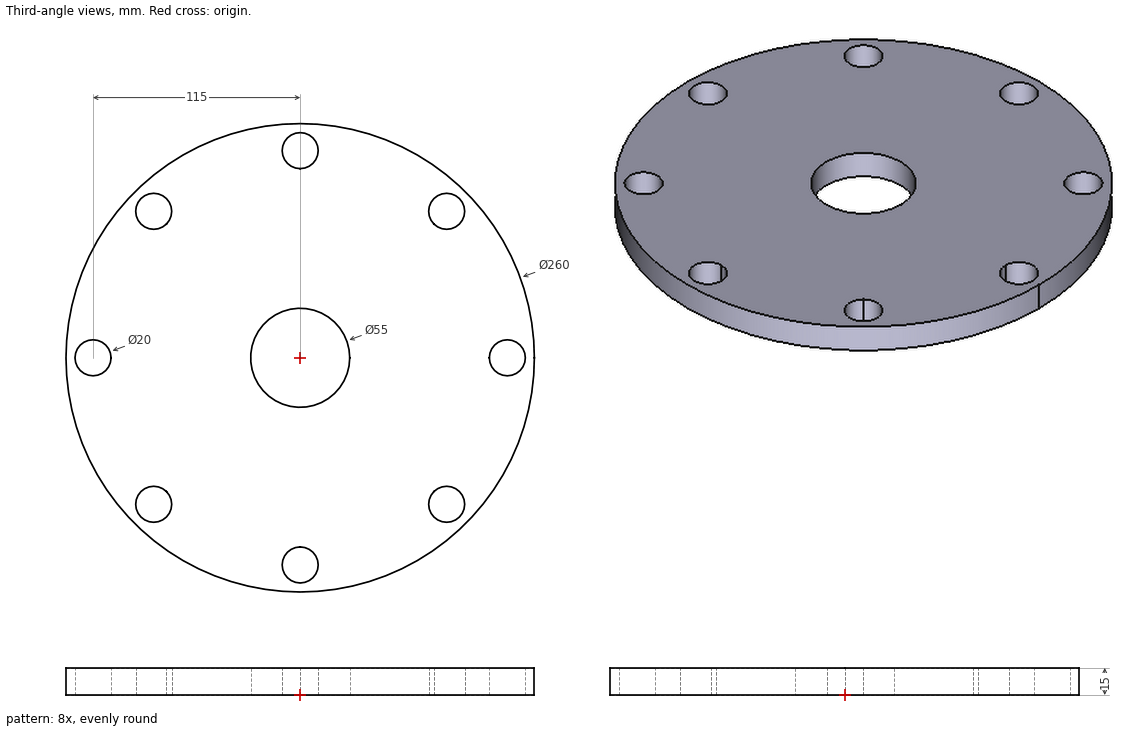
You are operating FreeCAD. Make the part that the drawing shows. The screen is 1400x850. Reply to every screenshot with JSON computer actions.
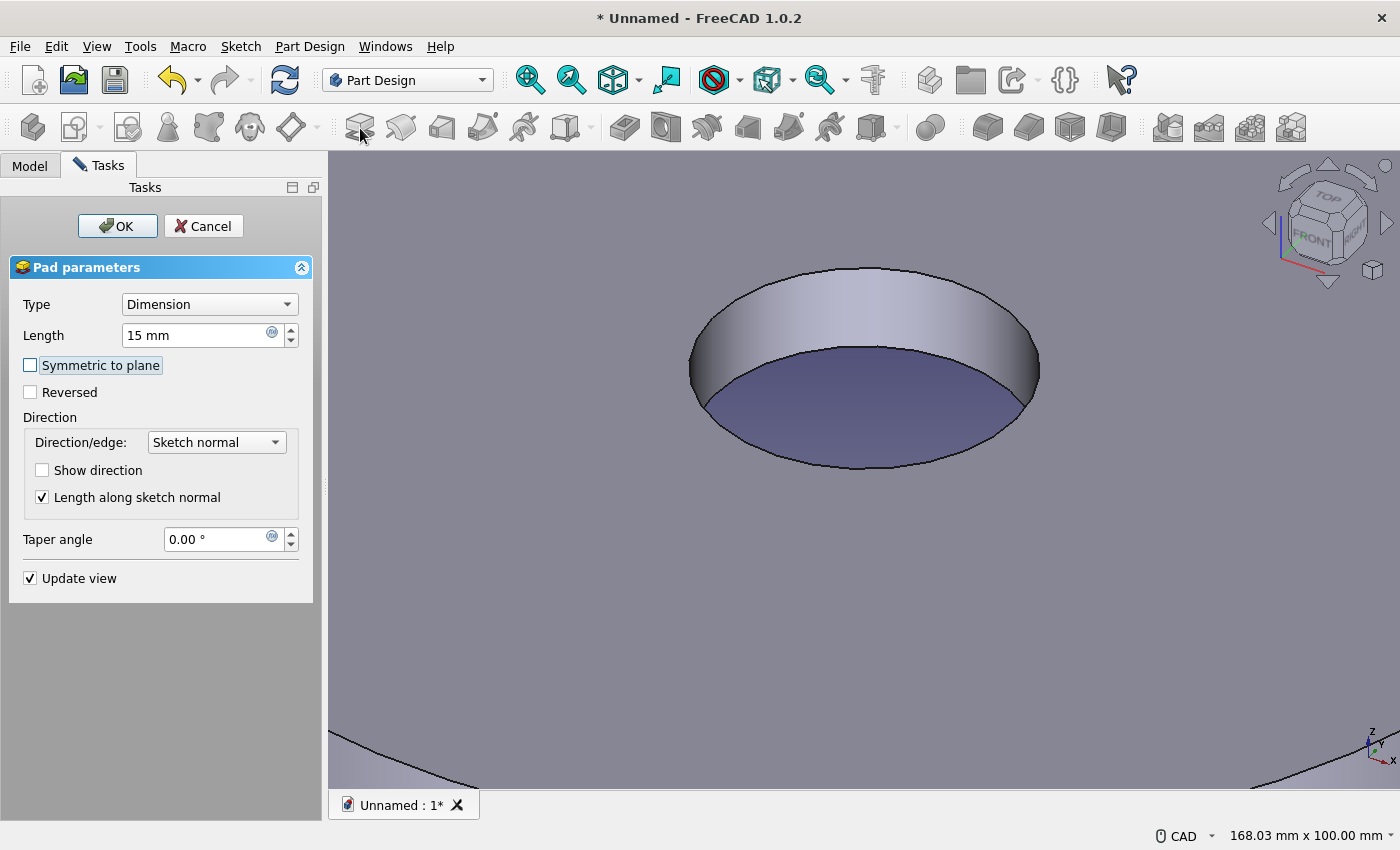
{"action": "left_click", "coordinate": [118, 226]}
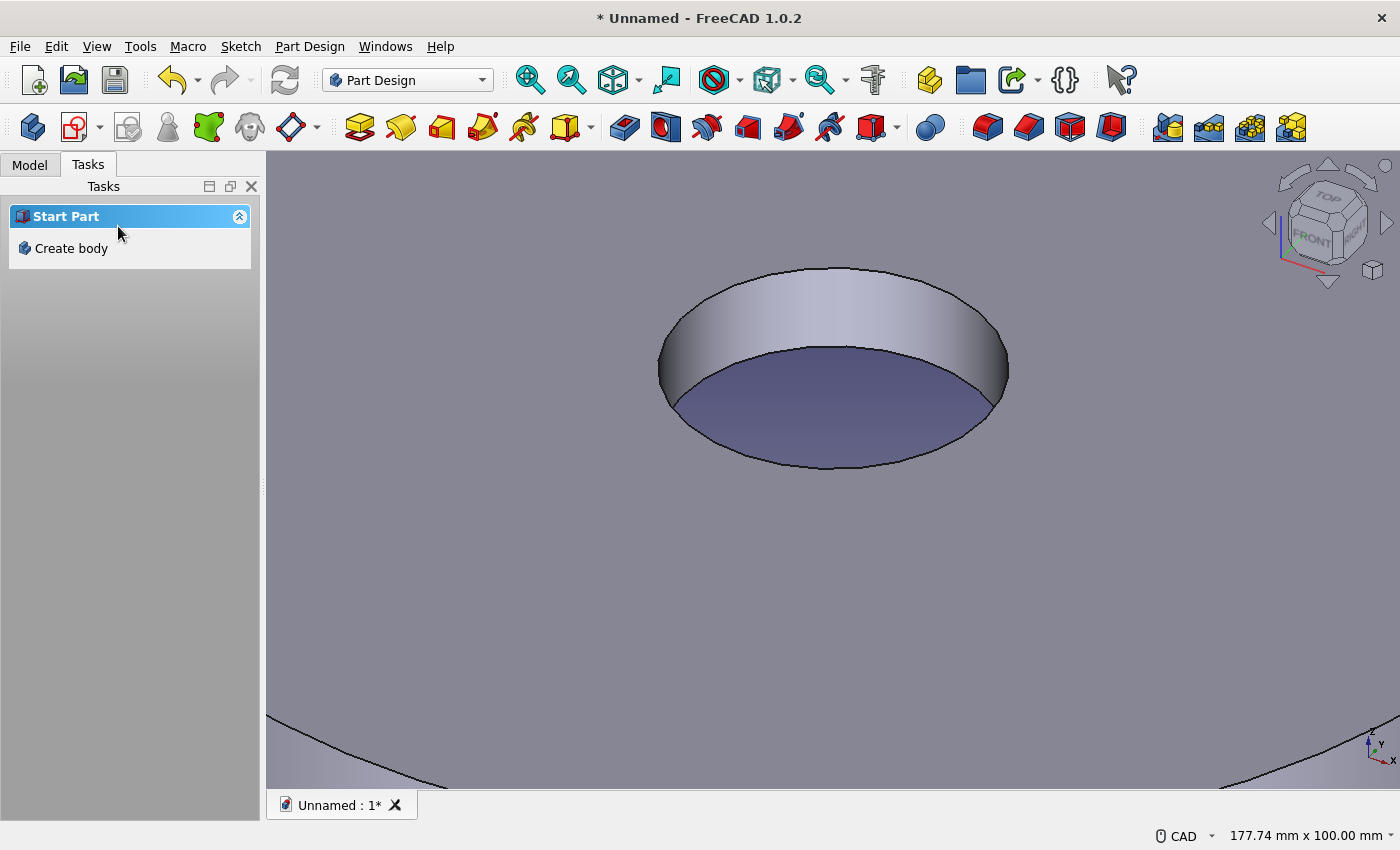
{"action": "left_click", "coordinate": [531, 80]}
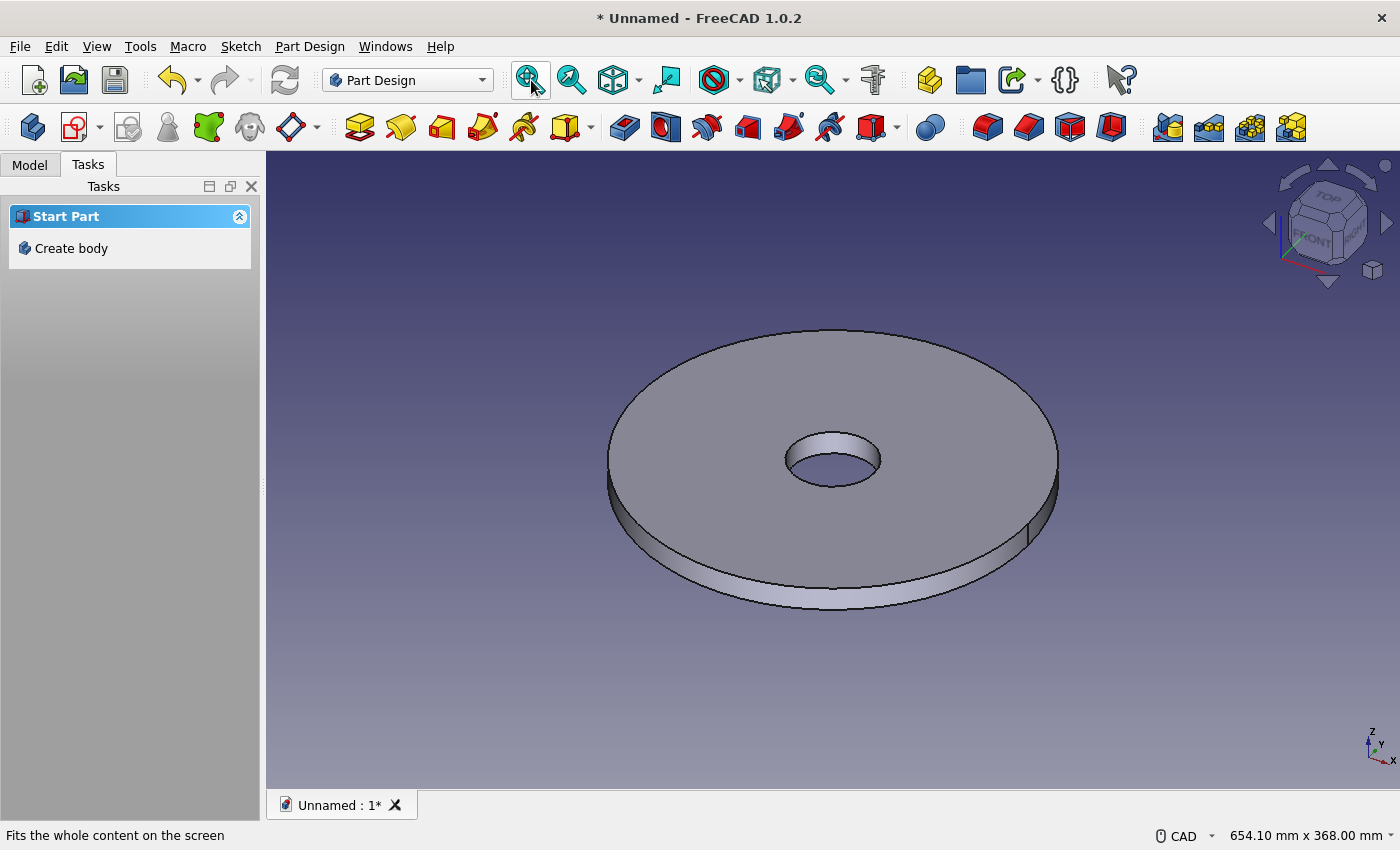
{"action": "key", "text": "5"}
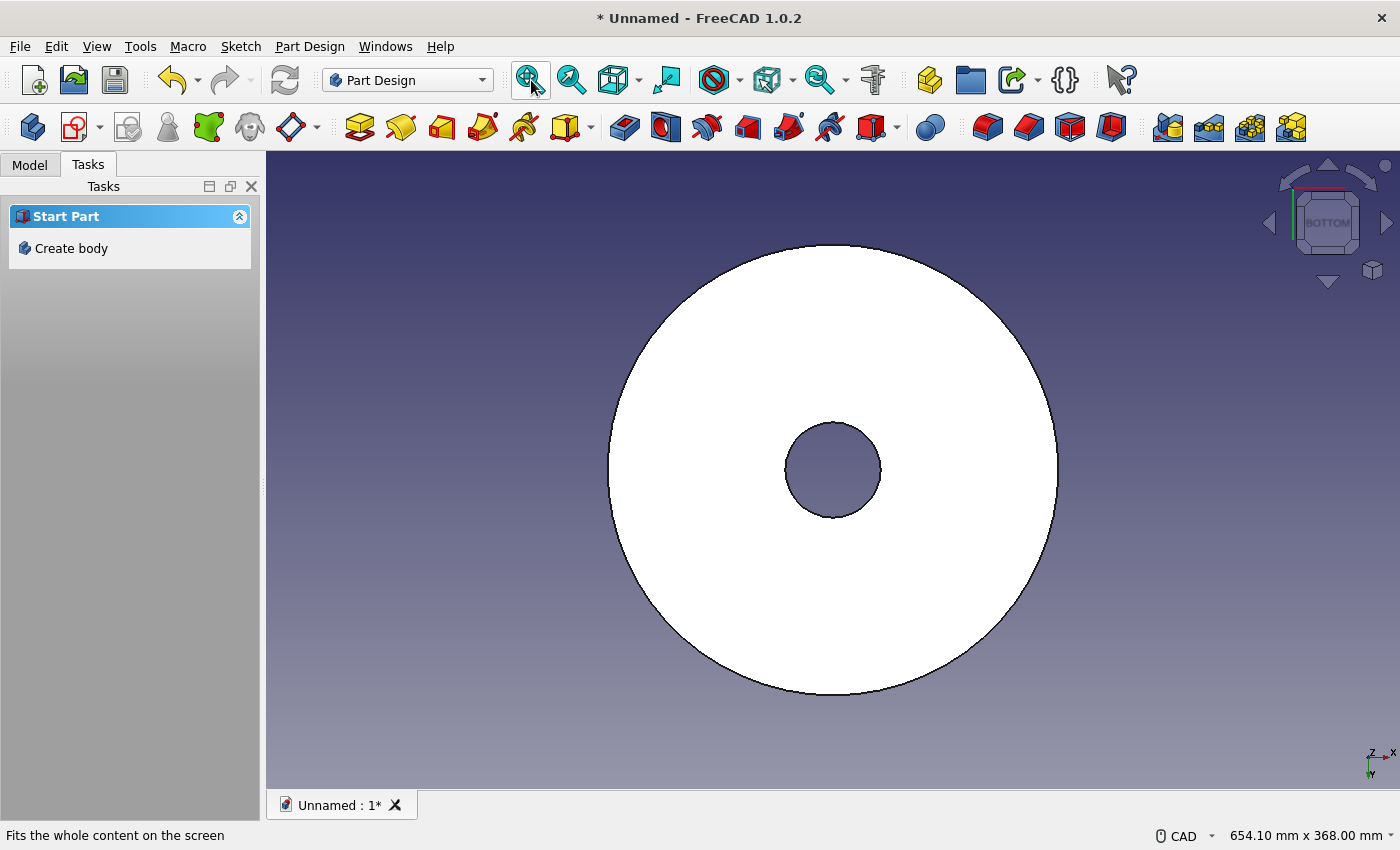
{"action": "left_click", "coordinate": [897, 598]}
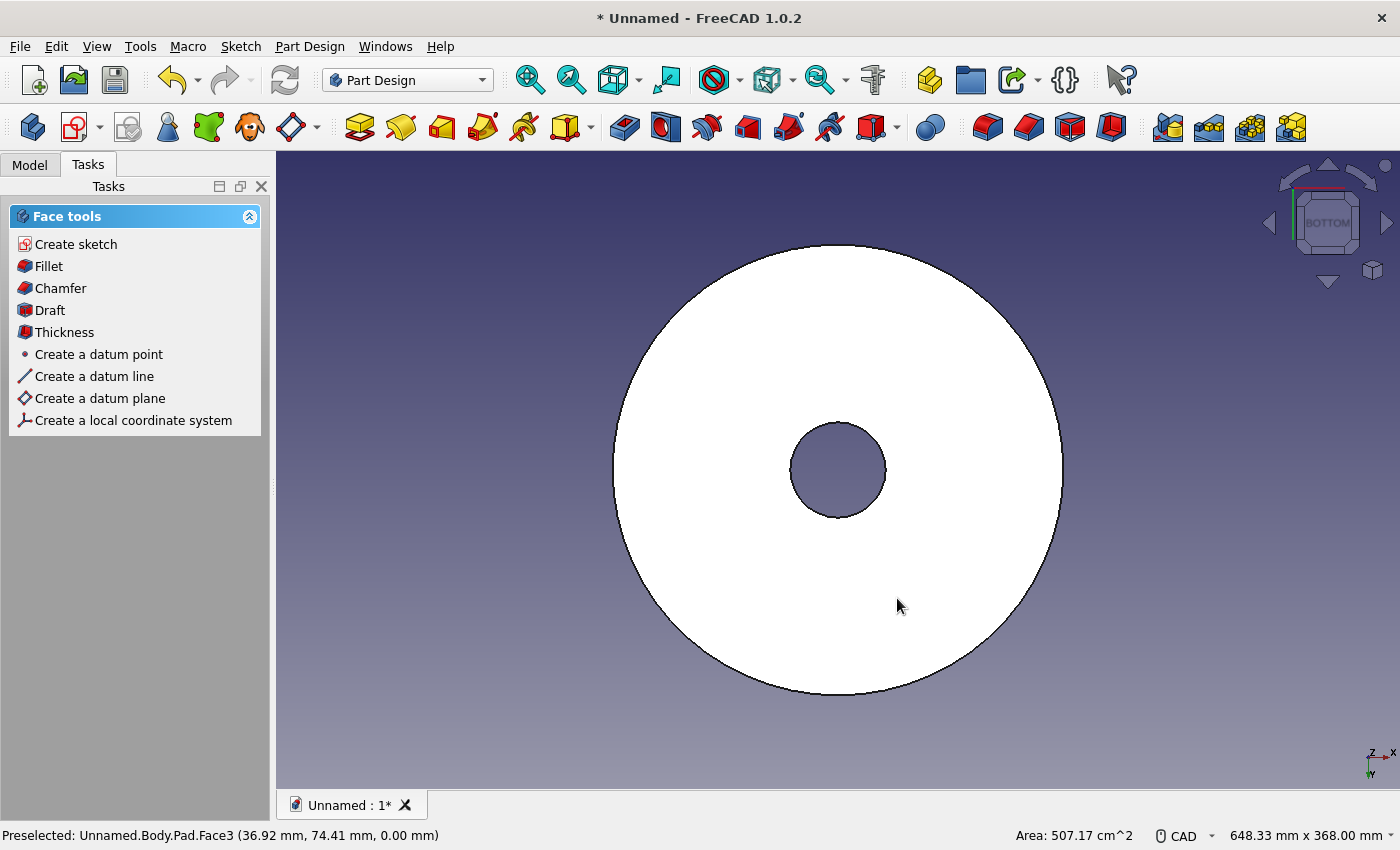
{"action": "left_click", "coordinate": [74, 128]}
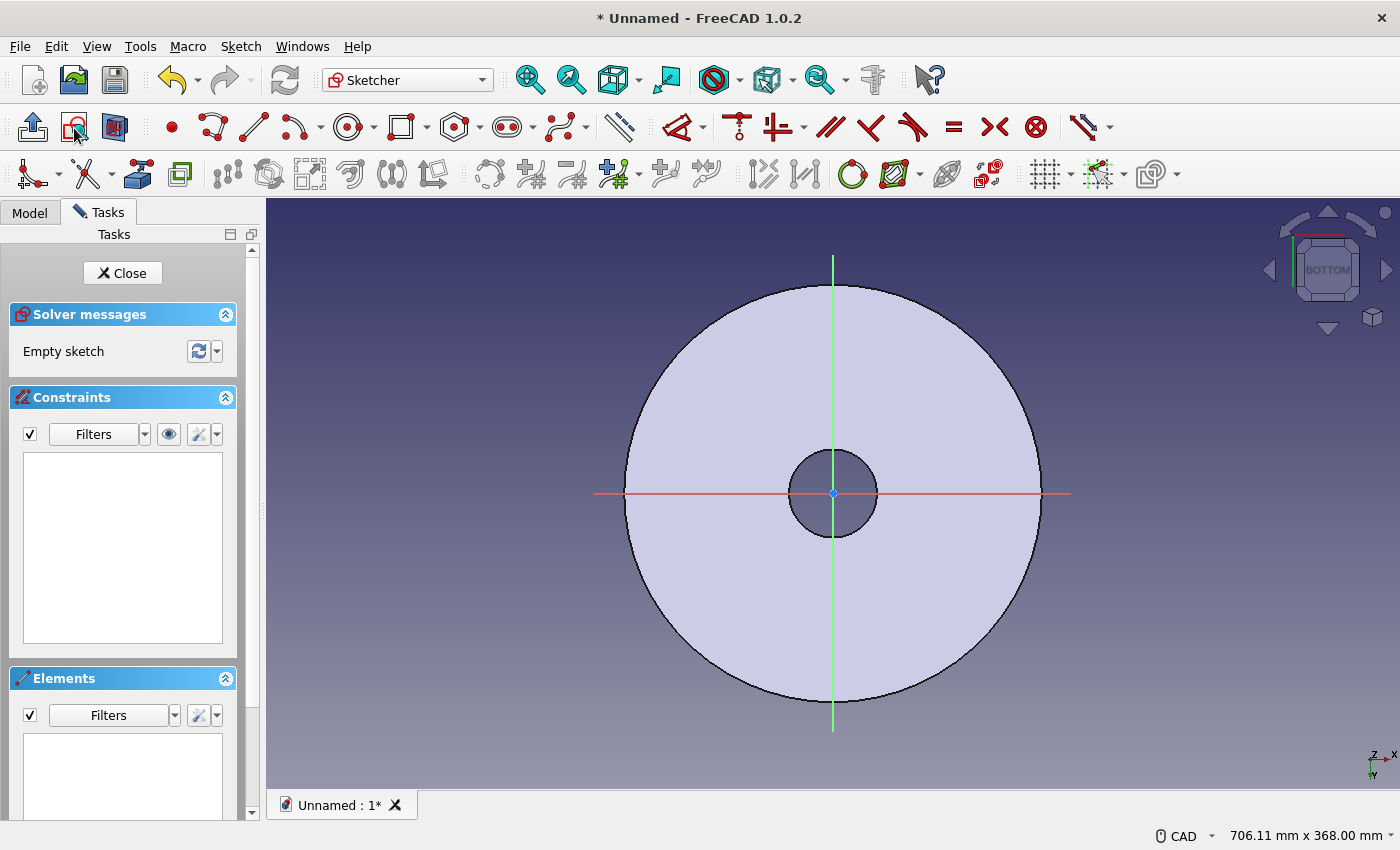
{"action": "scroll", "coordinate": [637, 494], "scroll_direction": "up", "scroll_amount": 12}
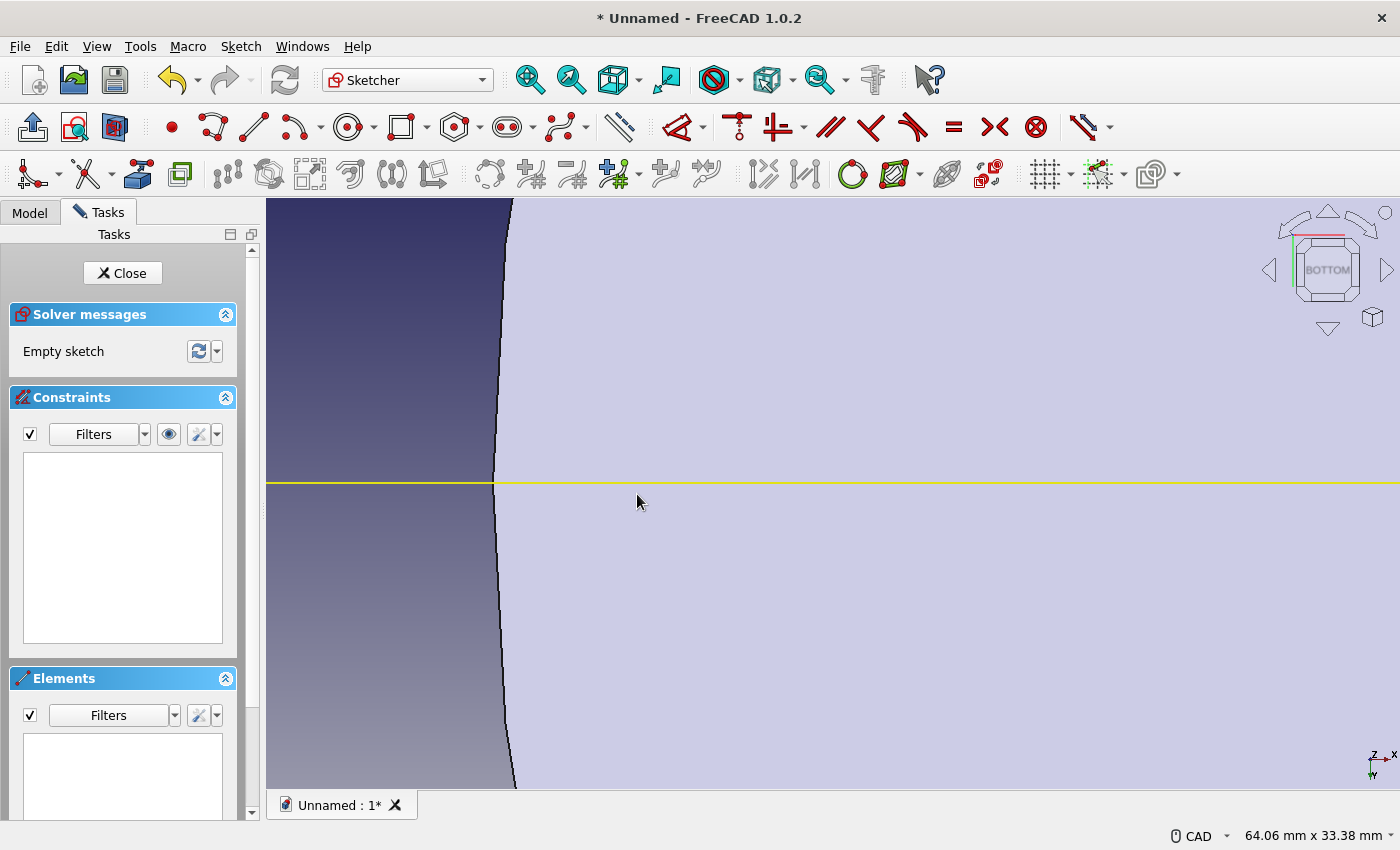
{"action": "left_click", "coordinate": [348, 128]}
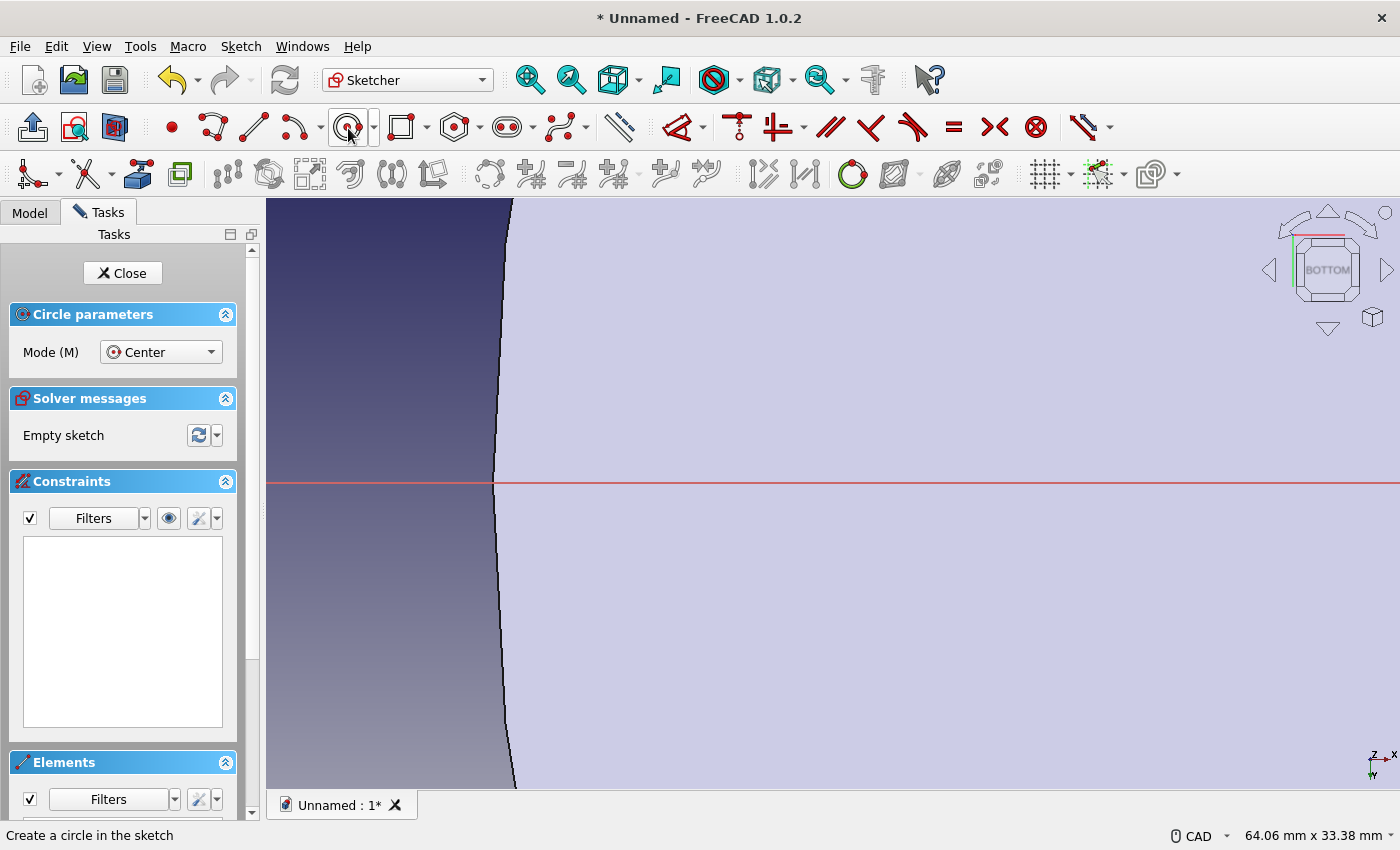
{"action": "left_click", "coordinate": [758, 483]}
{"action": "left_click", "coordinate": [884, 358]}
{"action": "key", "text": "Escape"}